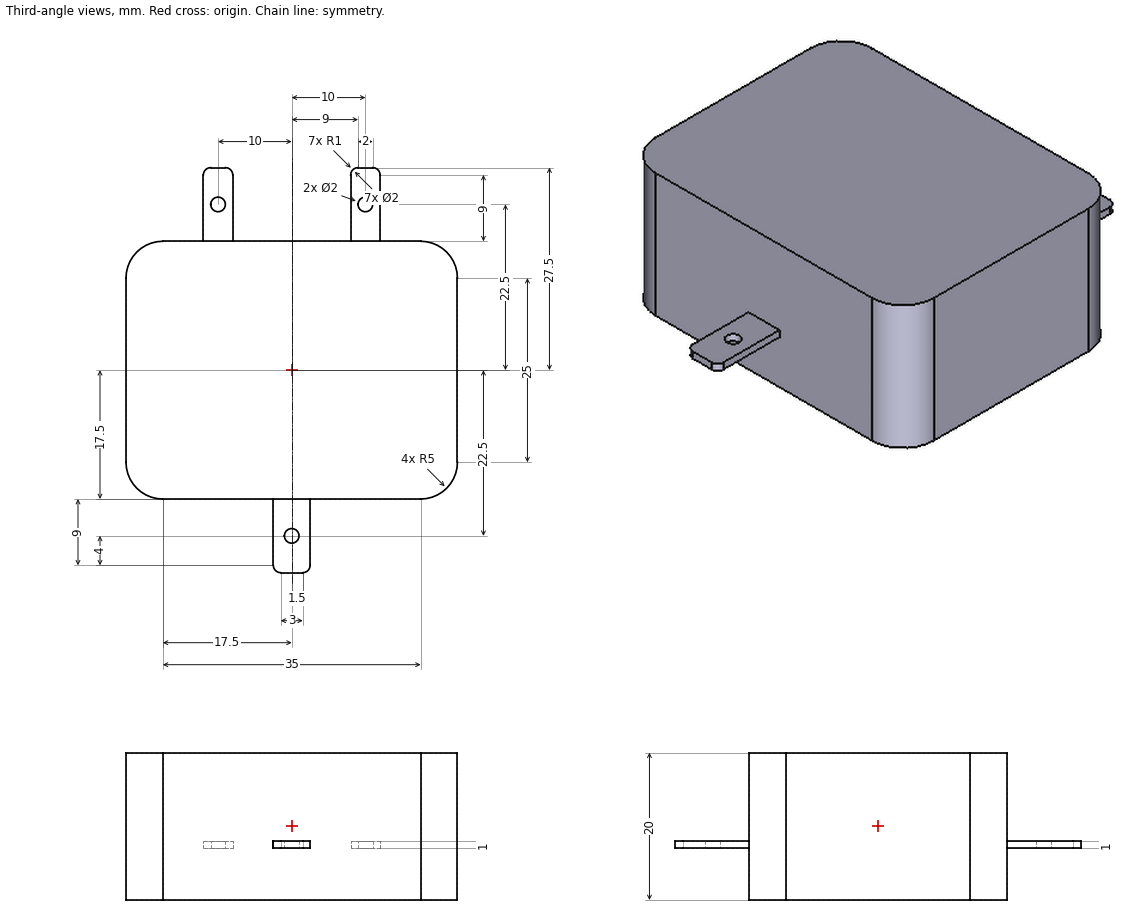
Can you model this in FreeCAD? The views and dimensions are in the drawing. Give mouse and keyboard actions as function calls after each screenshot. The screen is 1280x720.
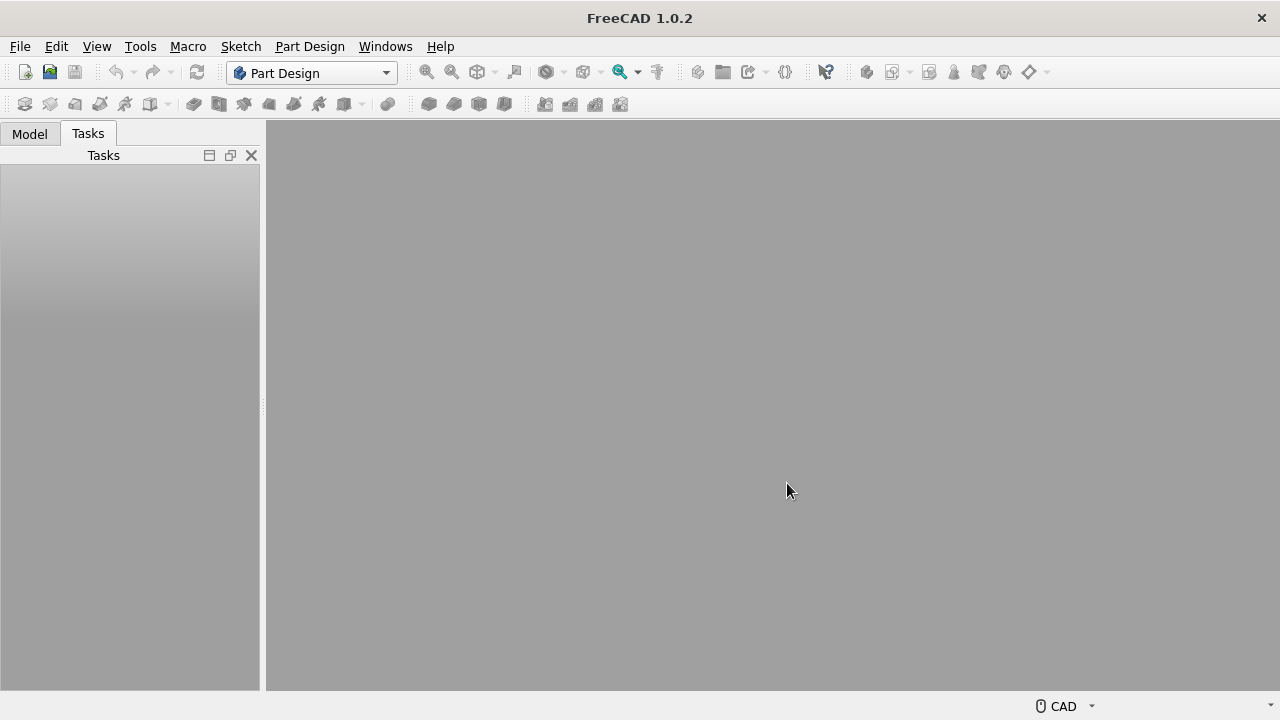
click(25, 72)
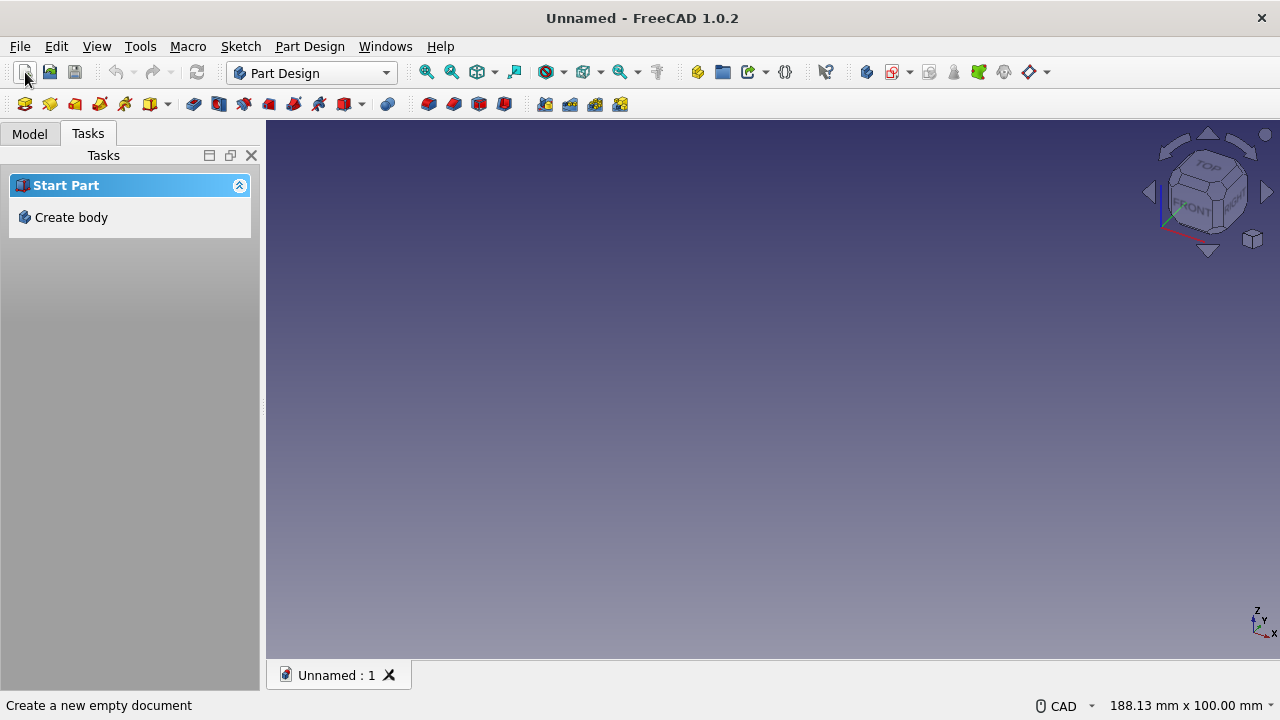
click(892, 72)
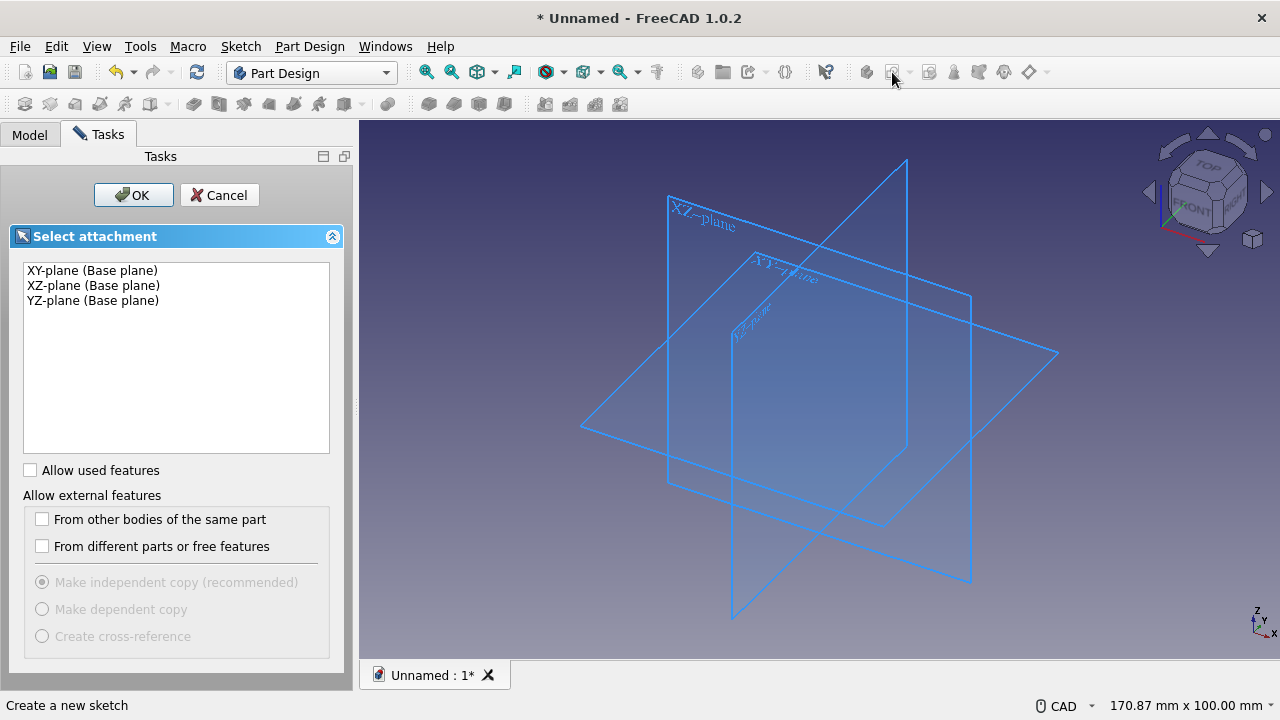
click(84, 270)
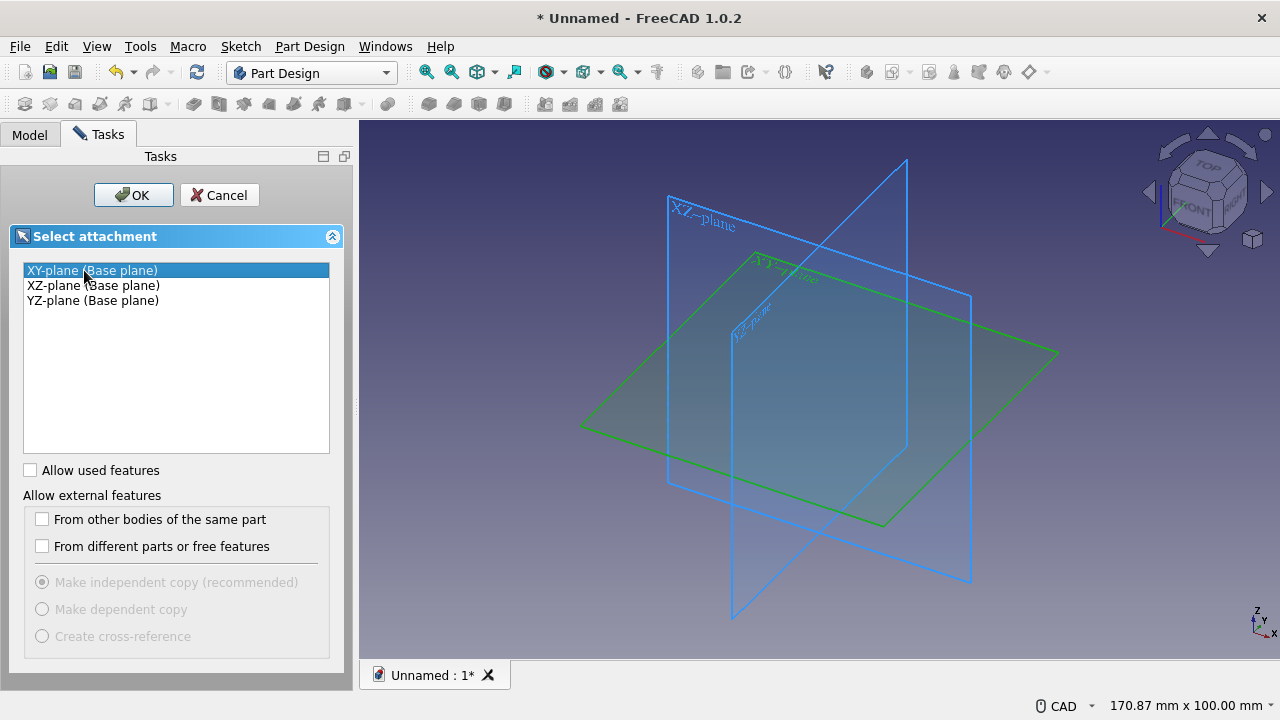
click(134, 195)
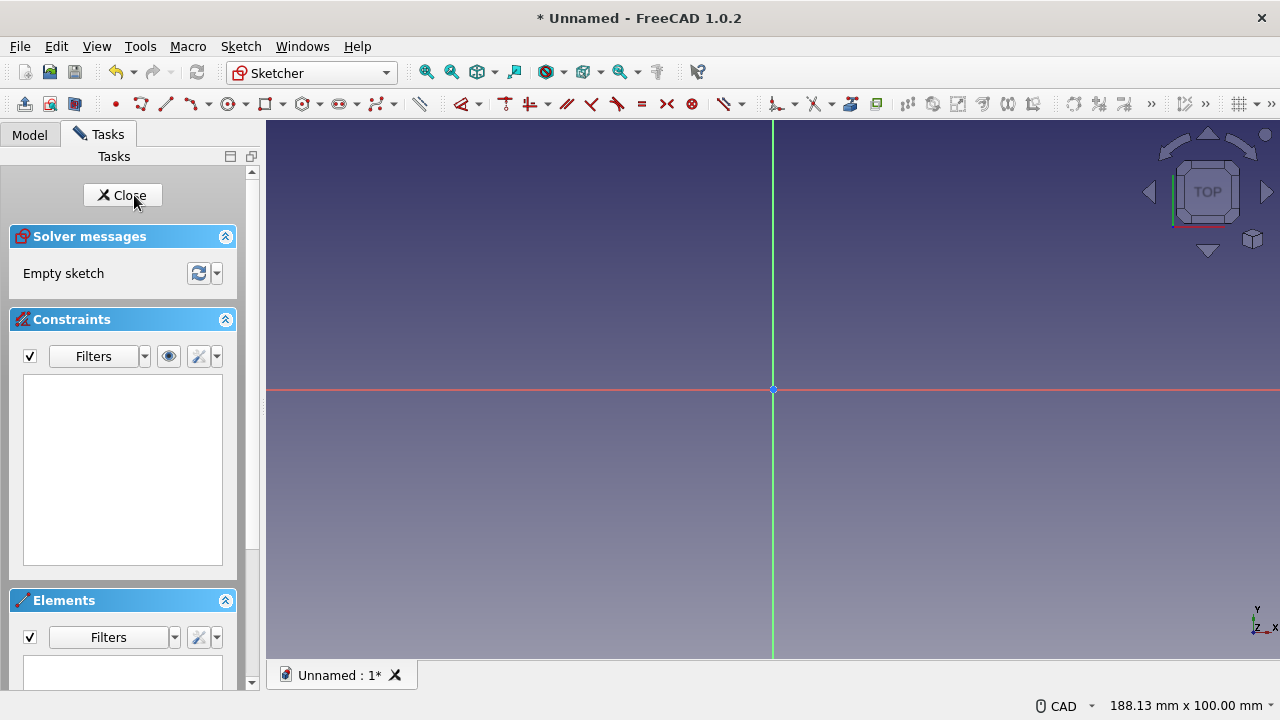
scroll(856, 389, up, 3)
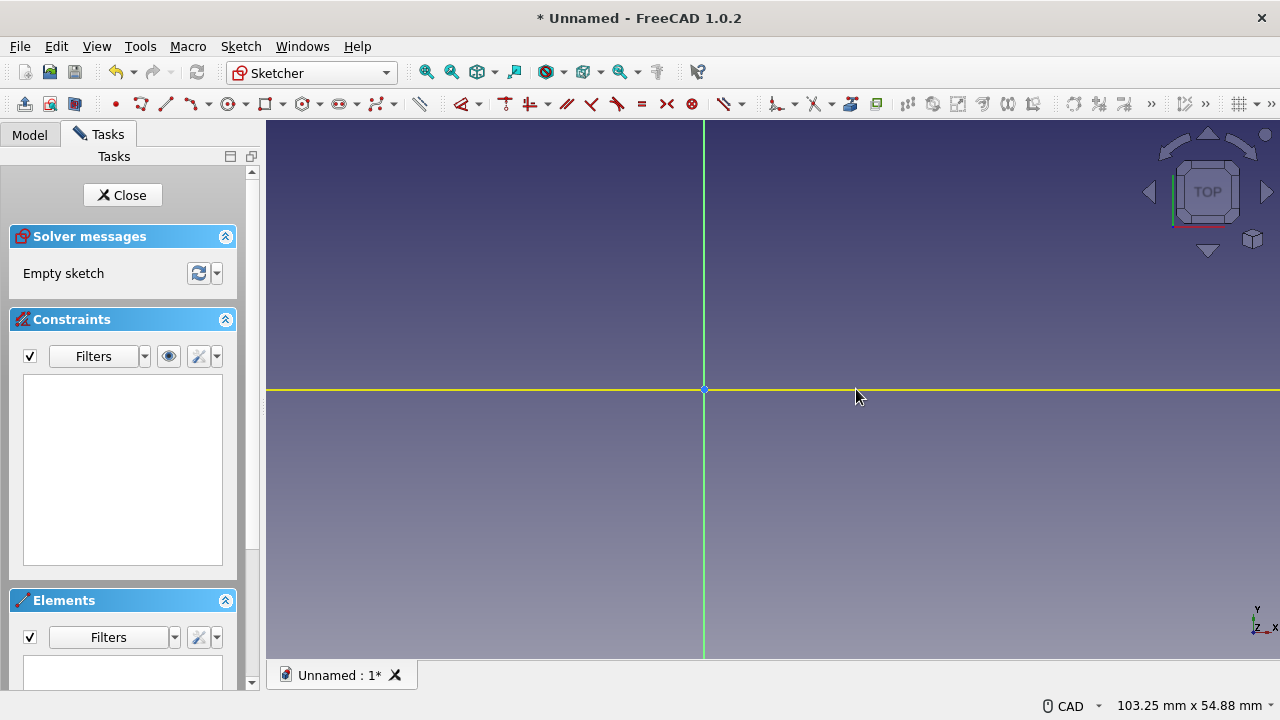
click(166, 104)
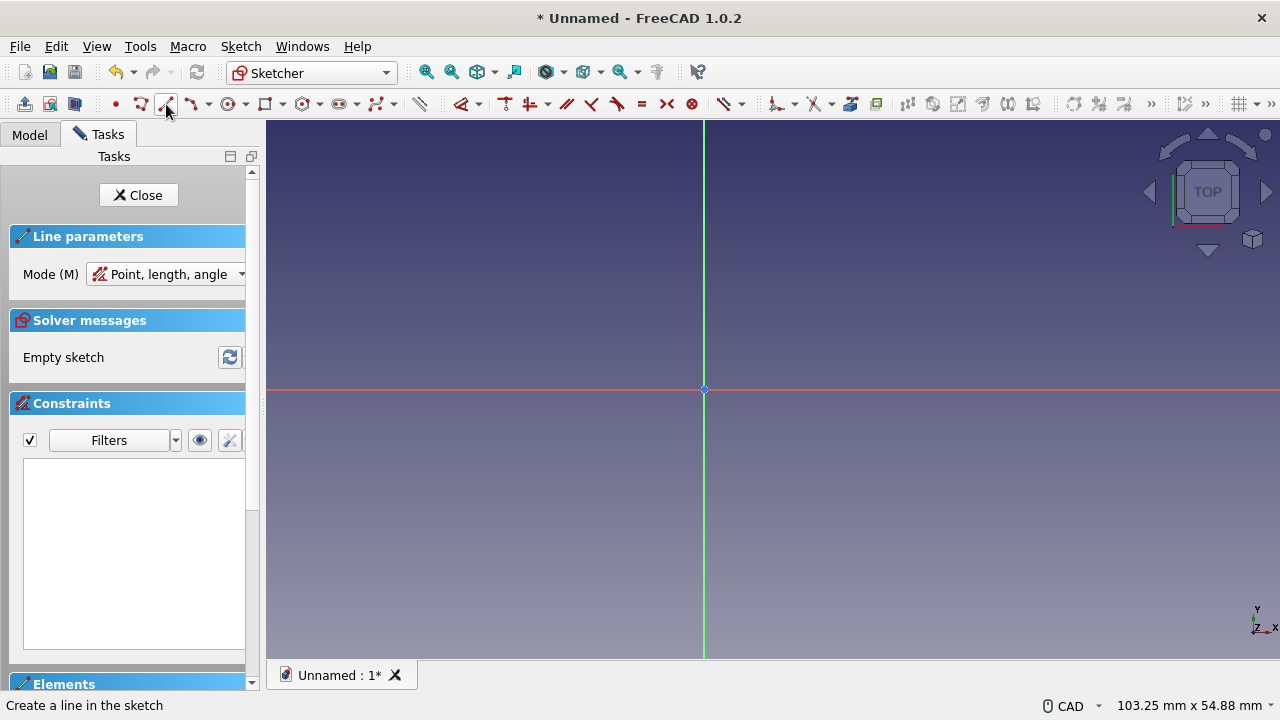
click(532, 561)
click(876, 561)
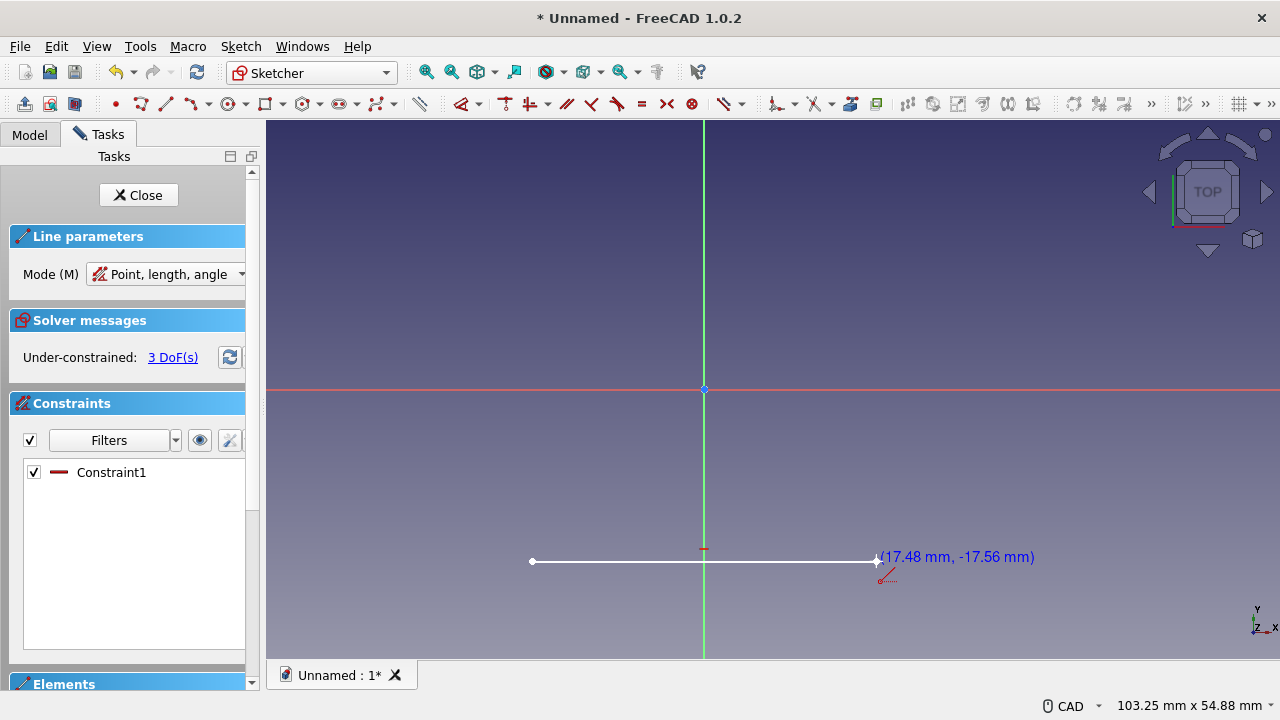
click(925, 512)
click(925, 267)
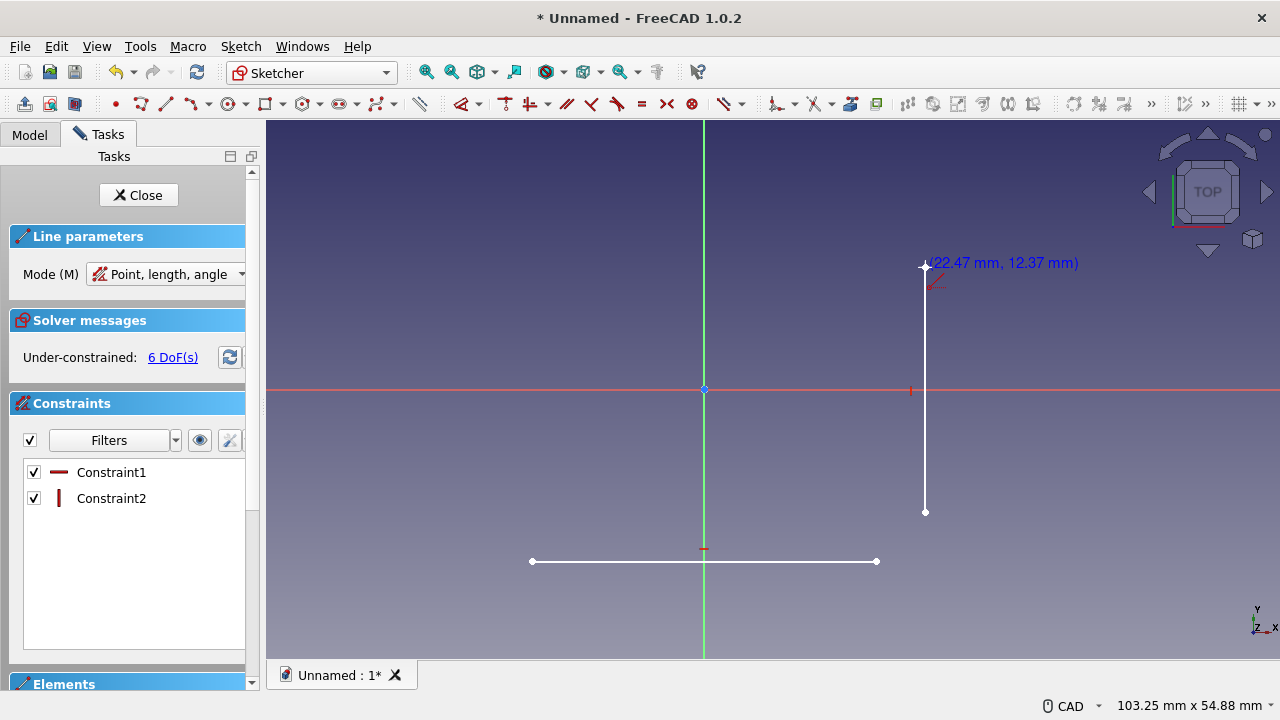
click(876, 218)
click(532, 218)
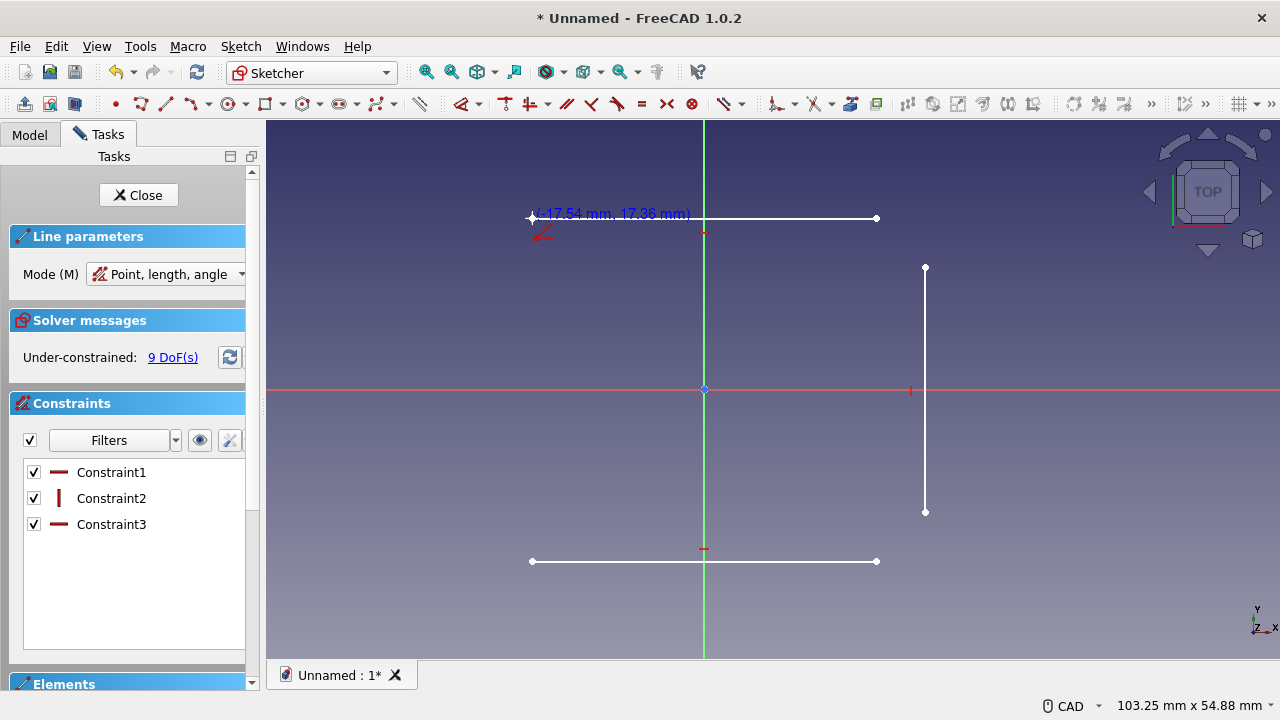
click(483, 267)
click(483, 512)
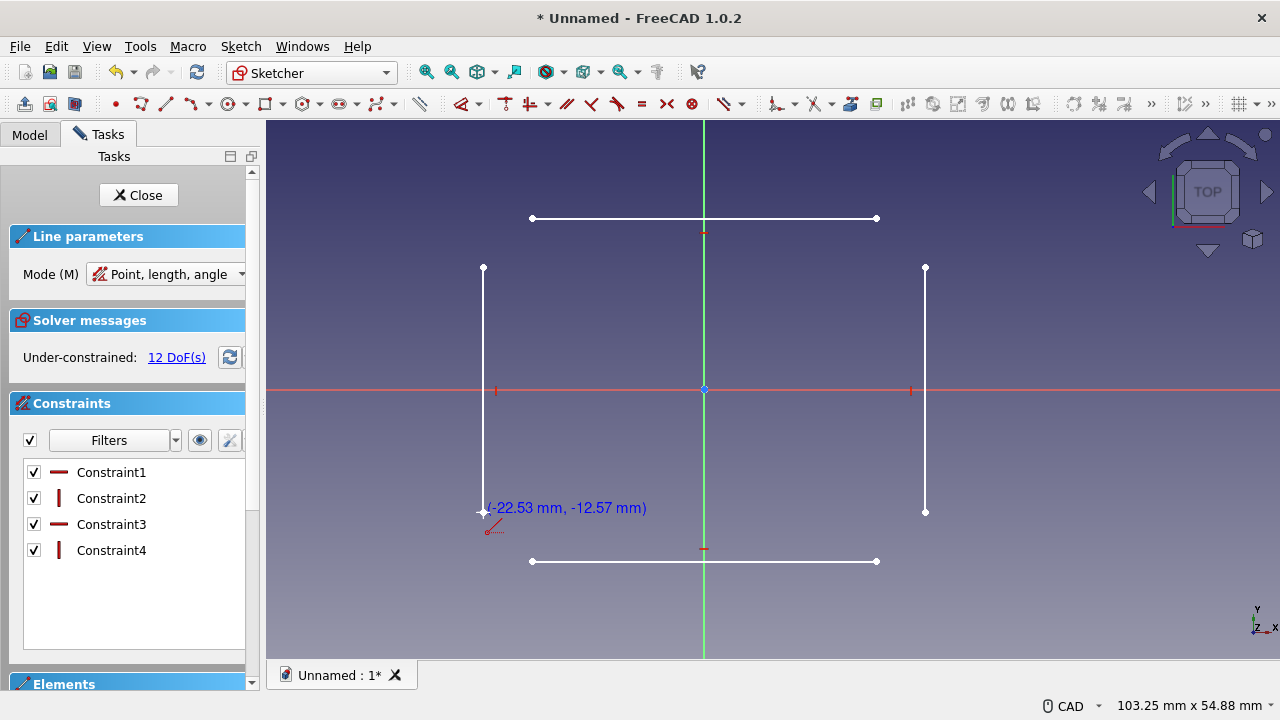
click(190, 104)